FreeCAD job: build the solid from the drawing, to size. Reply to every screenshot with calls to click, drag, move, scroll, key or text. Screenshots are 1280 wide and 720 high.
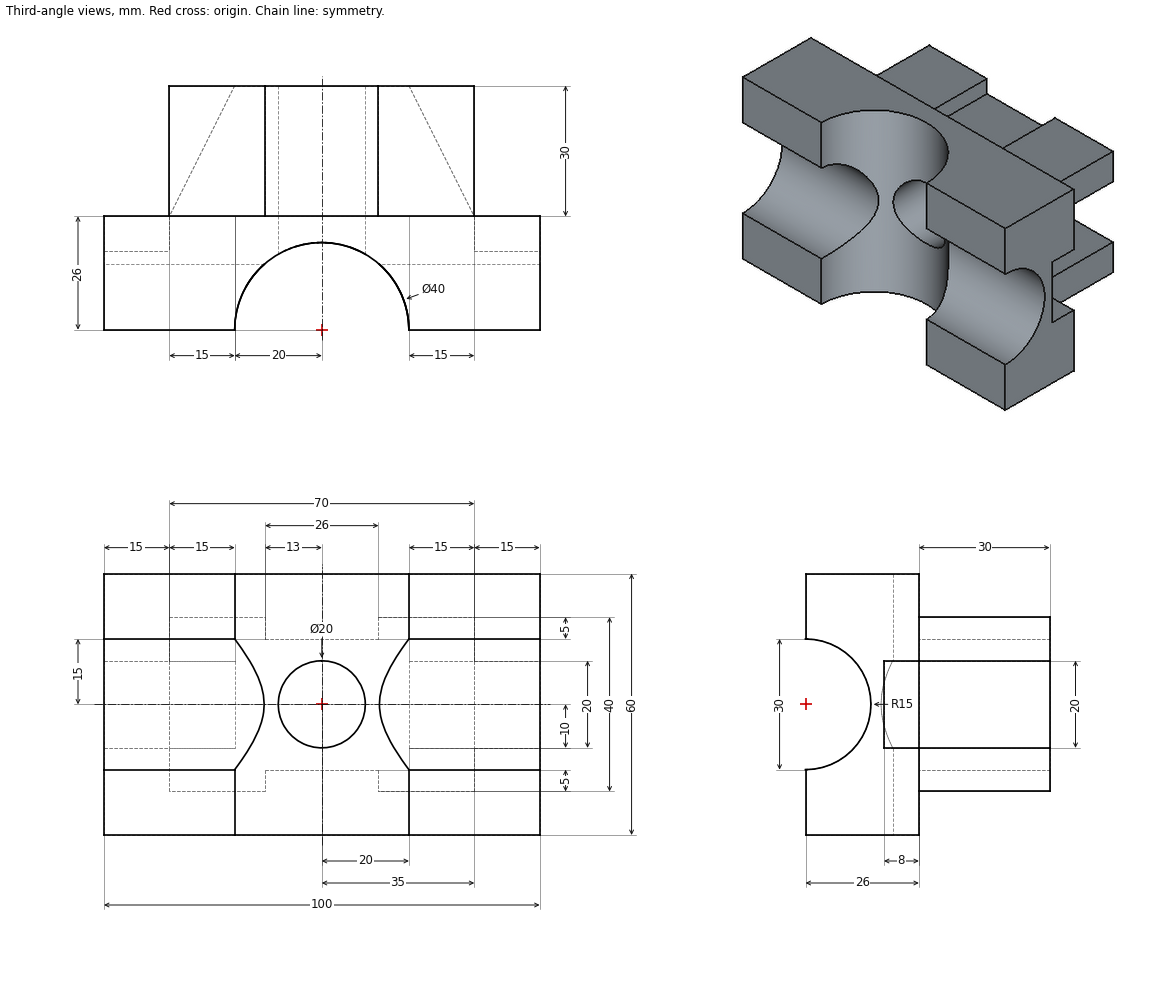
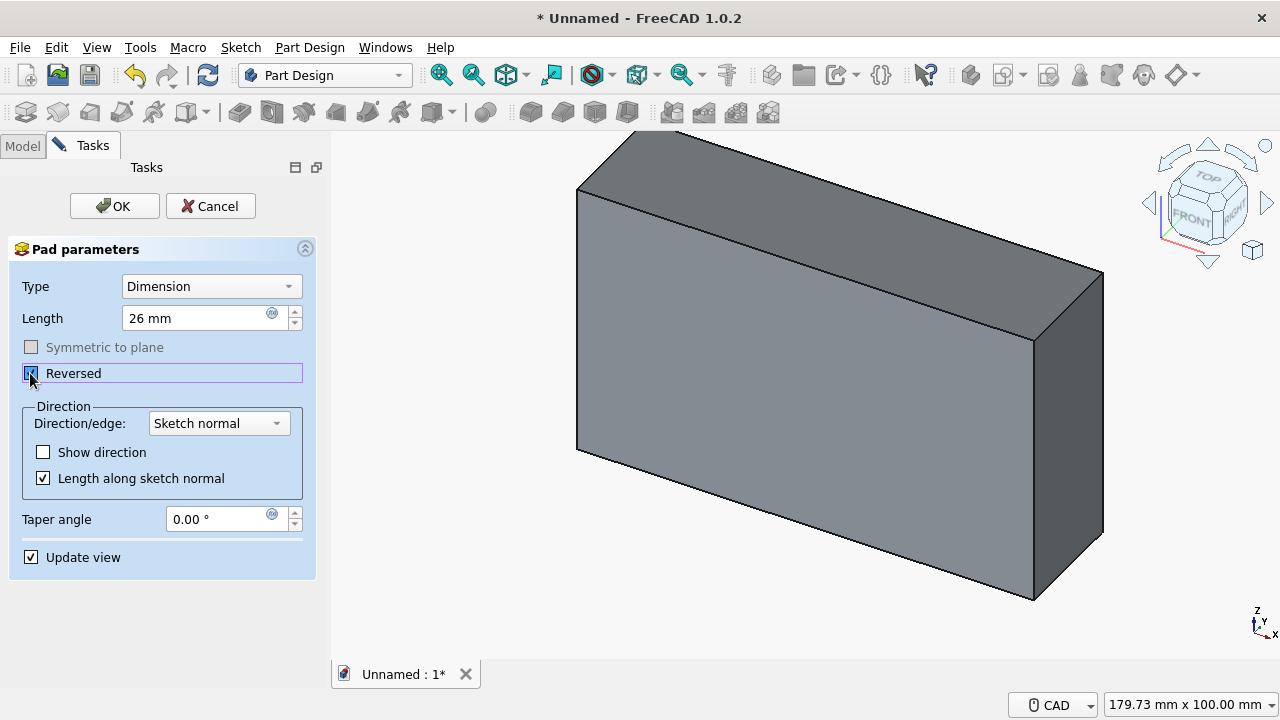
click(115, 206)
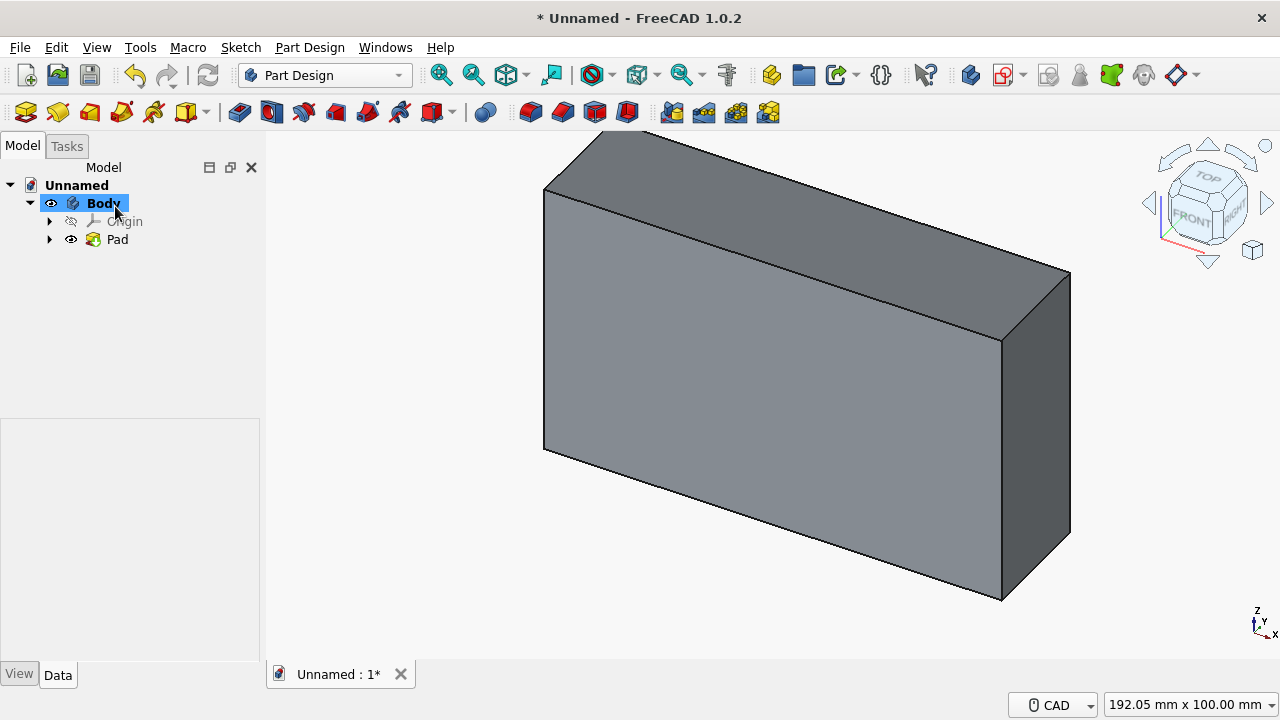
click(442, 76)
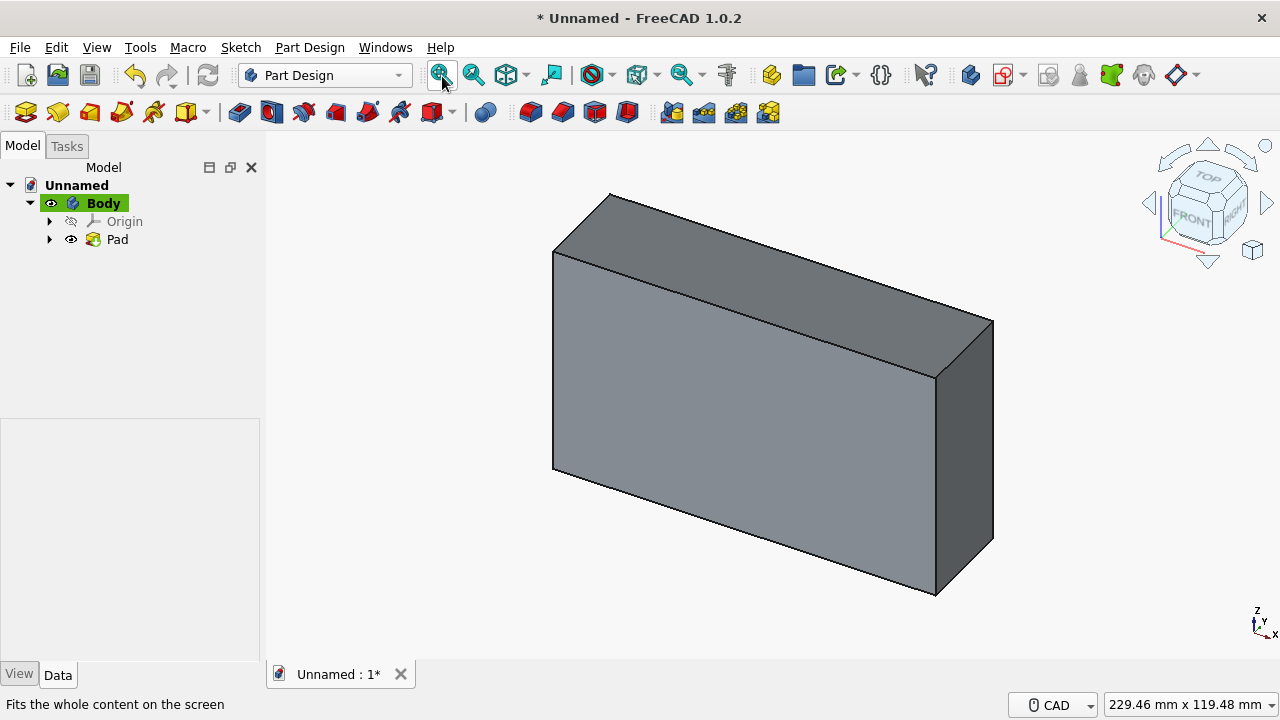
key(4)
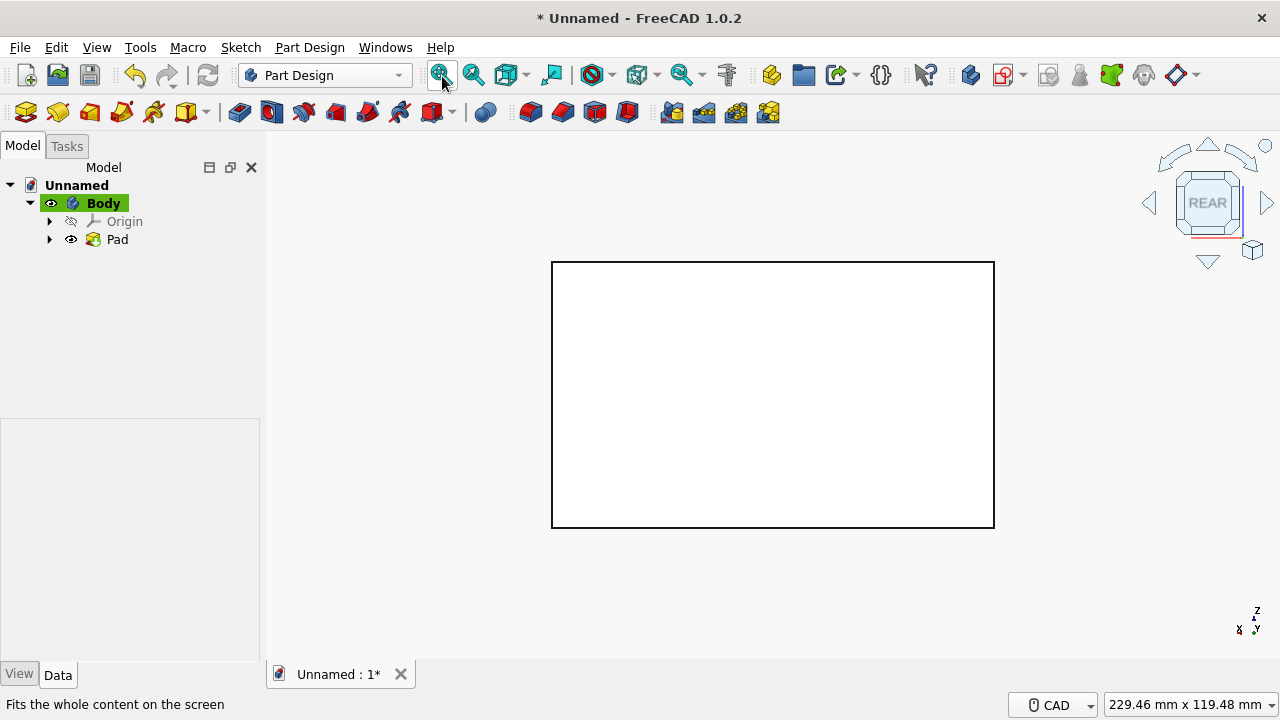
click(710, 394)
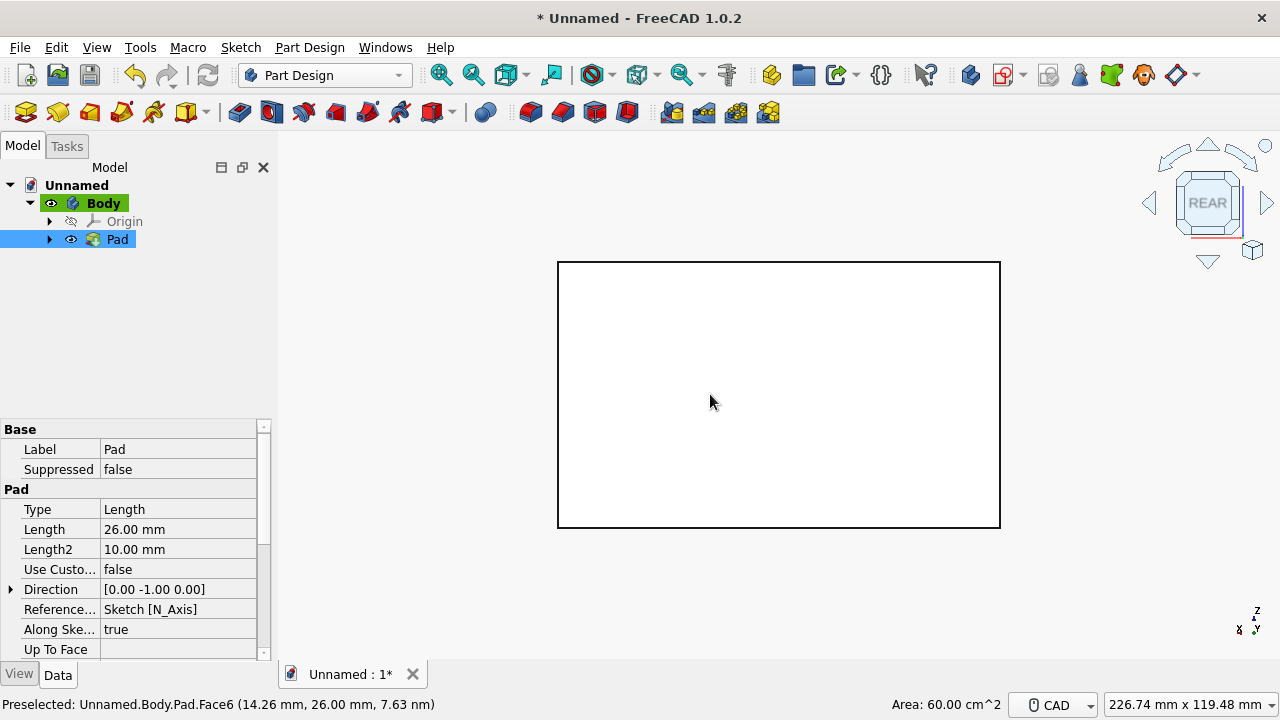
click(1004, 76)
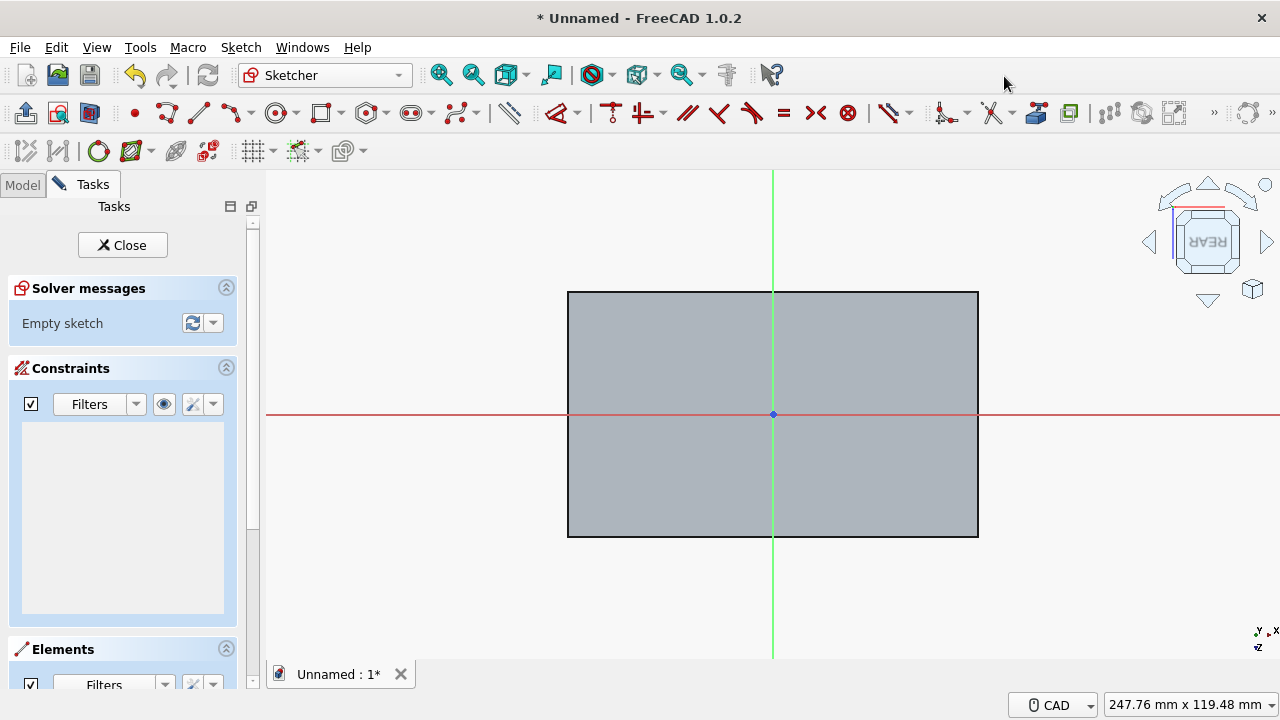
scroll(856, 414, up, 3)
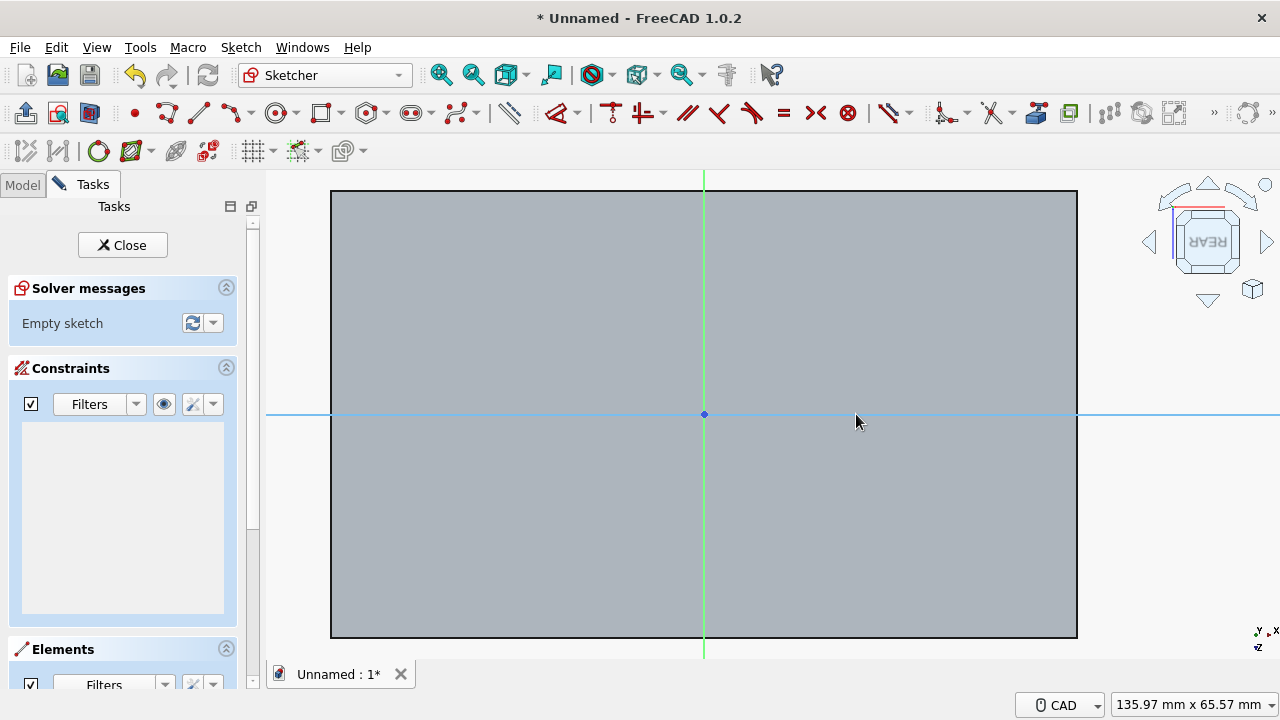
key(g)
key(v)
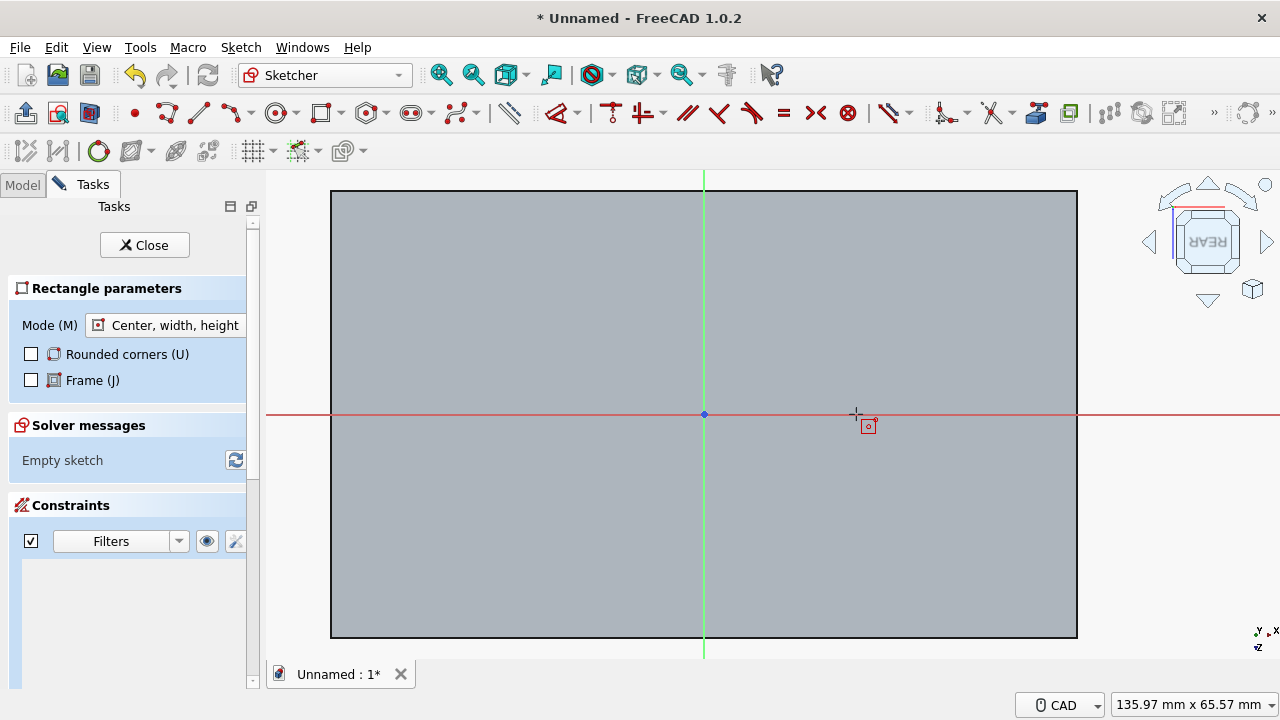
click(704, 414)
move(965, 265)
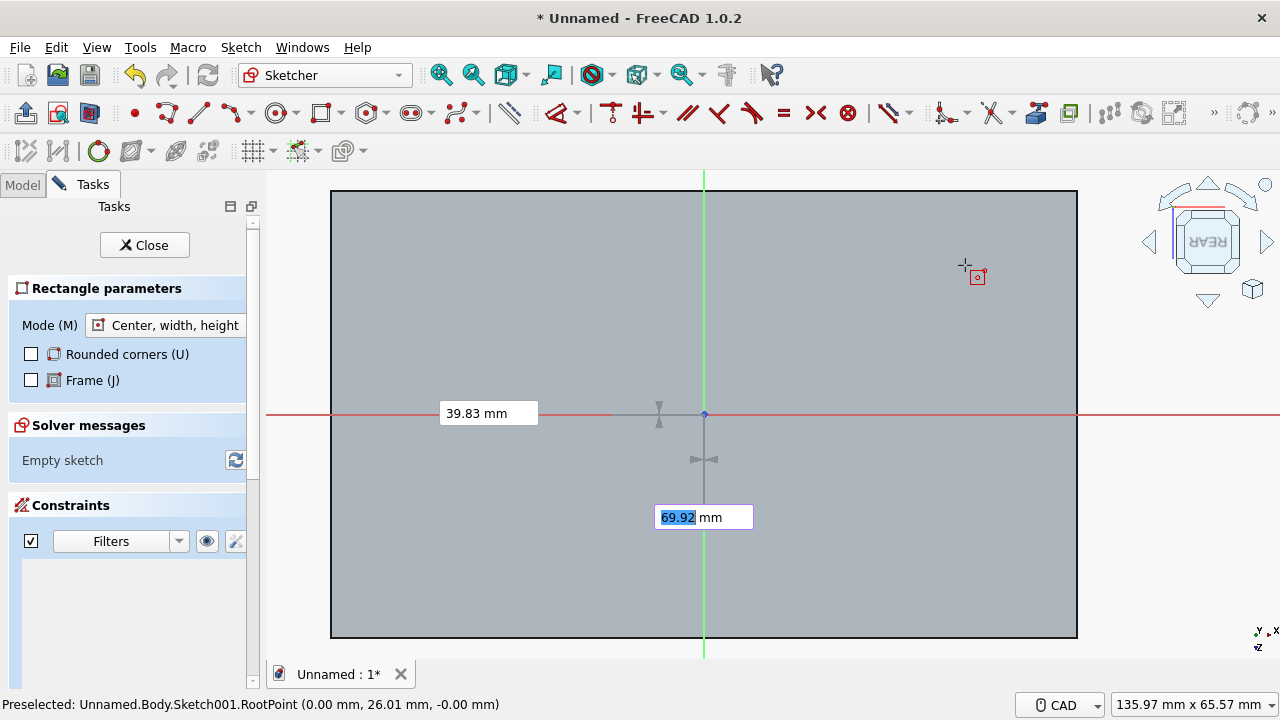
text(70)
key(Tab)
text(40)
key(Return)
key(Escape)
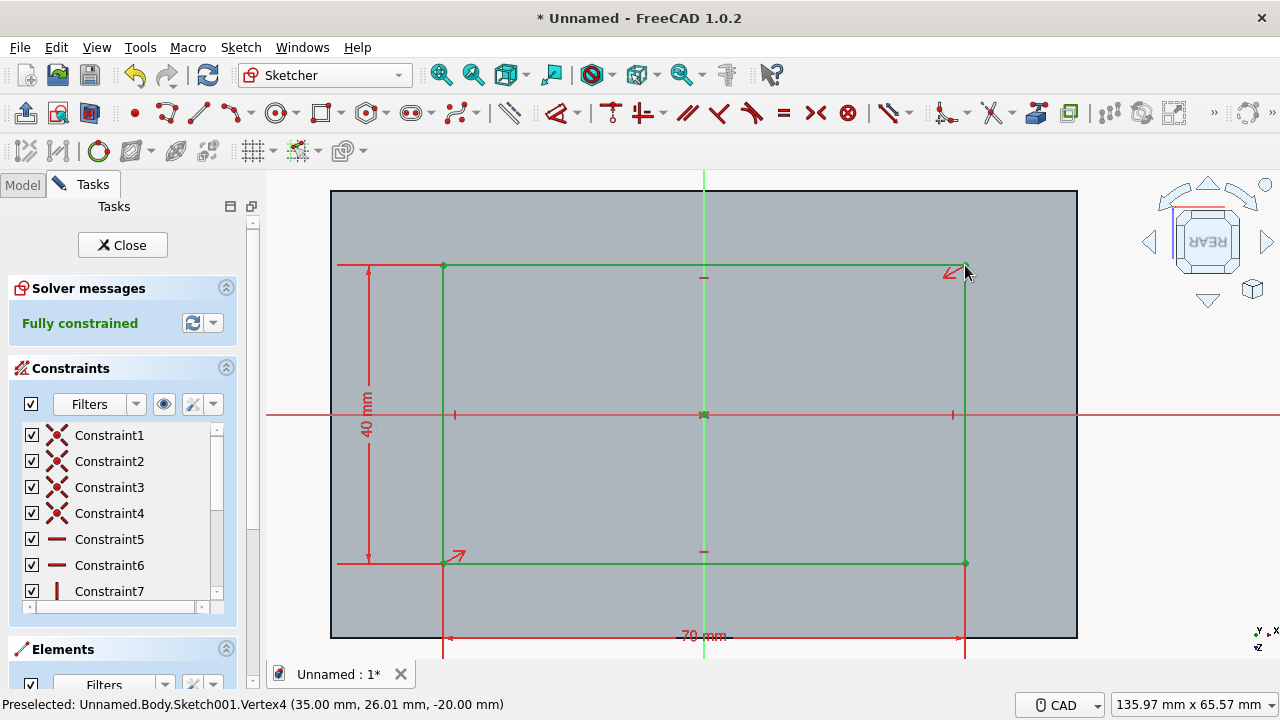
click(123, 245)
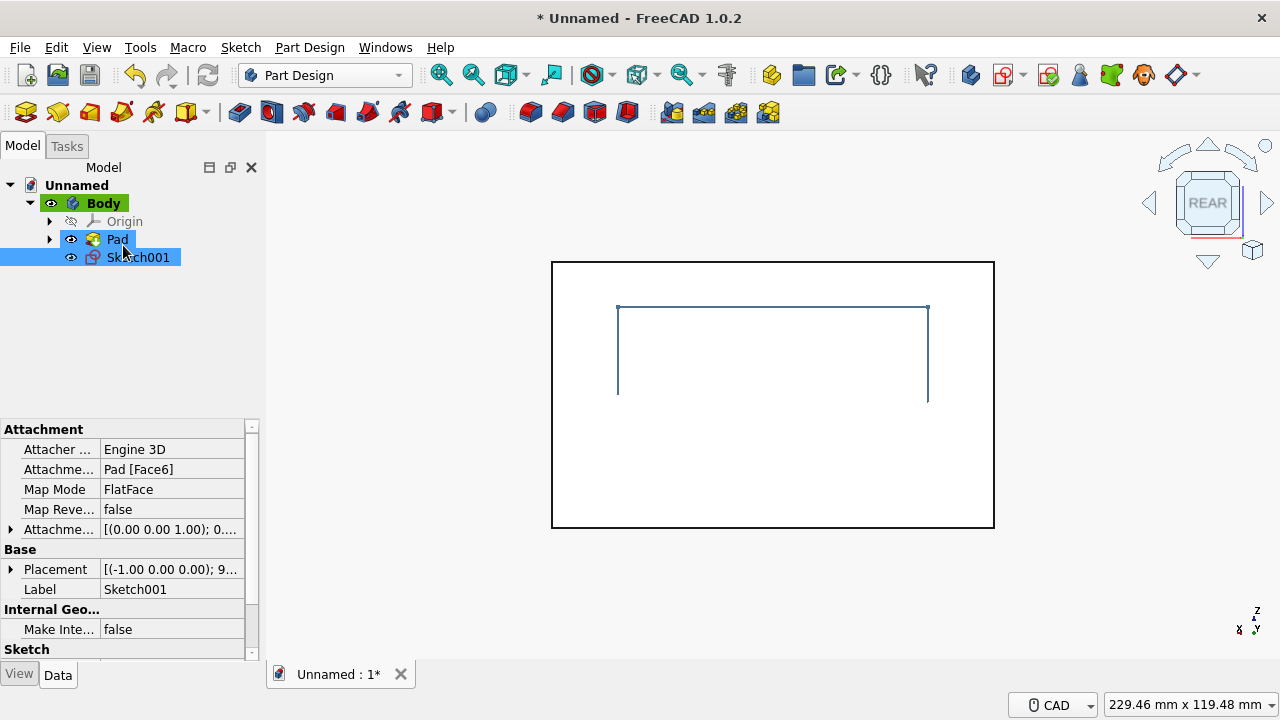
click(26, 112)